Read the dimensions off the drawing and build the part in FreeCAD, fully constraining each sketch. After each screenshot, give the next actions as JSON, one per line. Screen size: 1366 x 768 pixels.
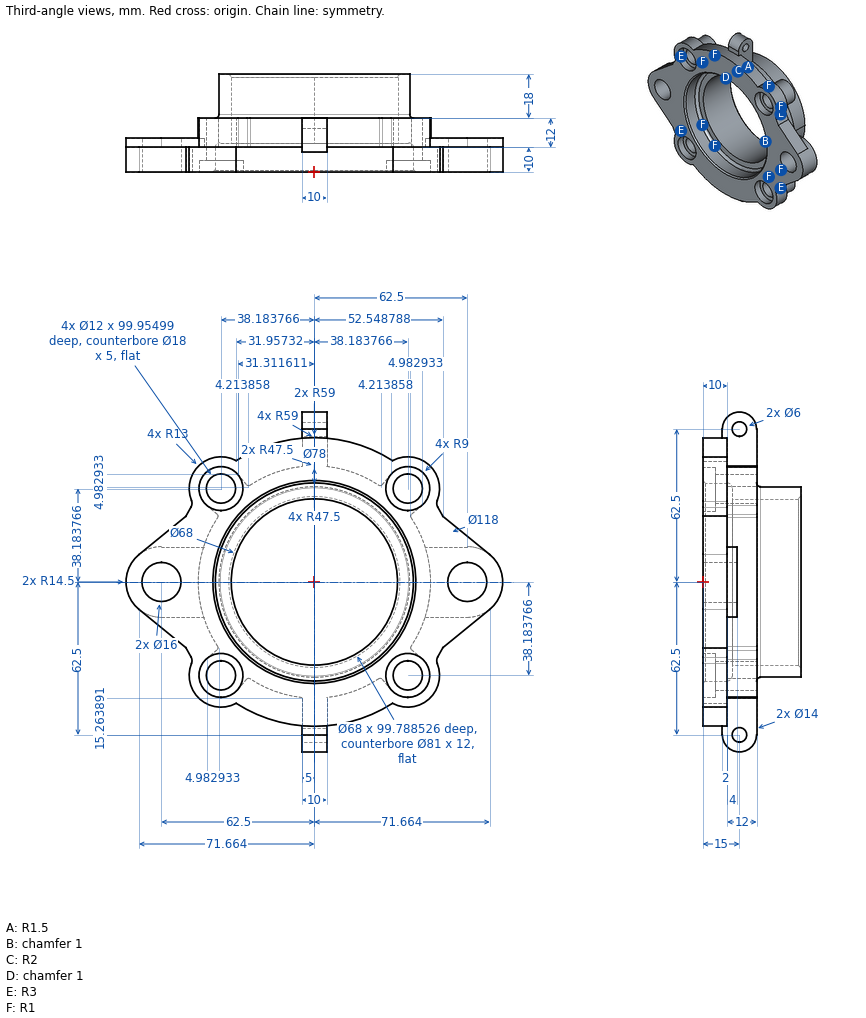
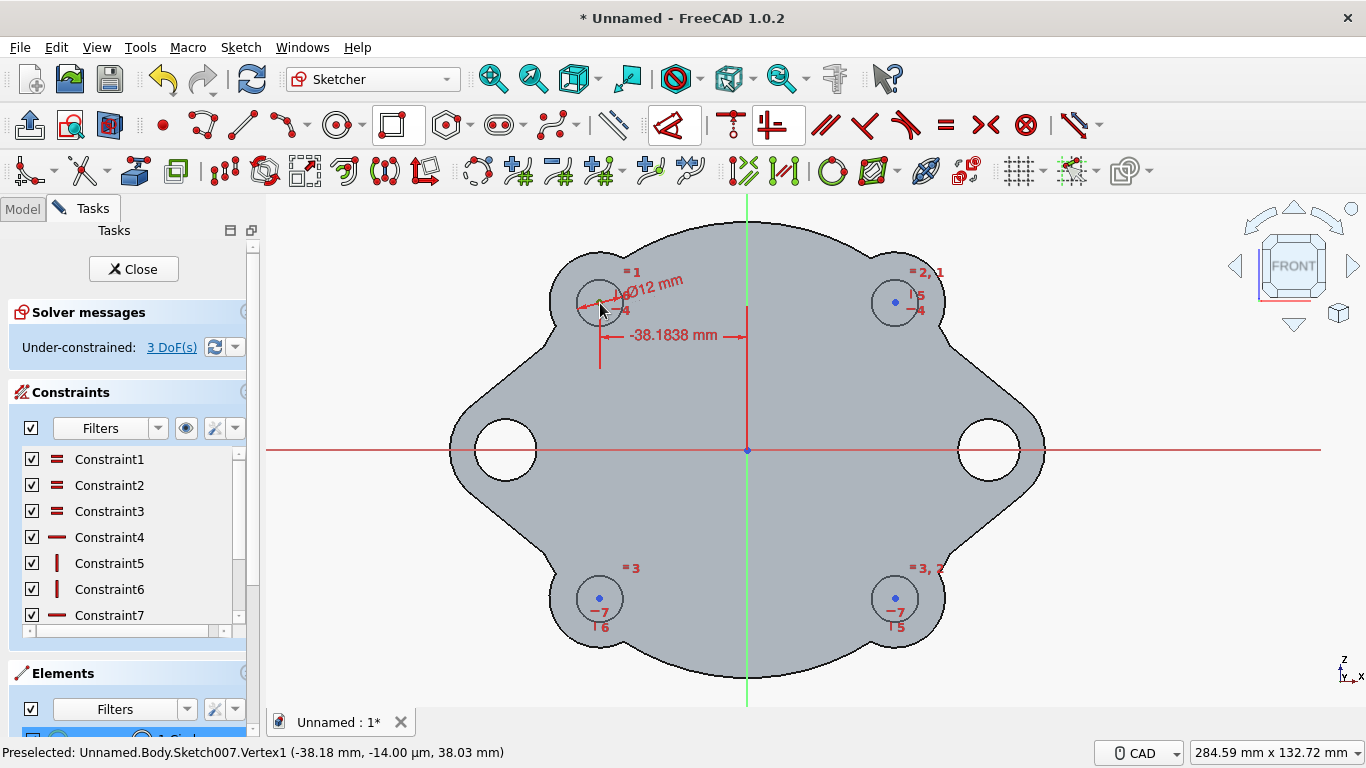
{"action": "left_click", "coordinate": [696, 126]}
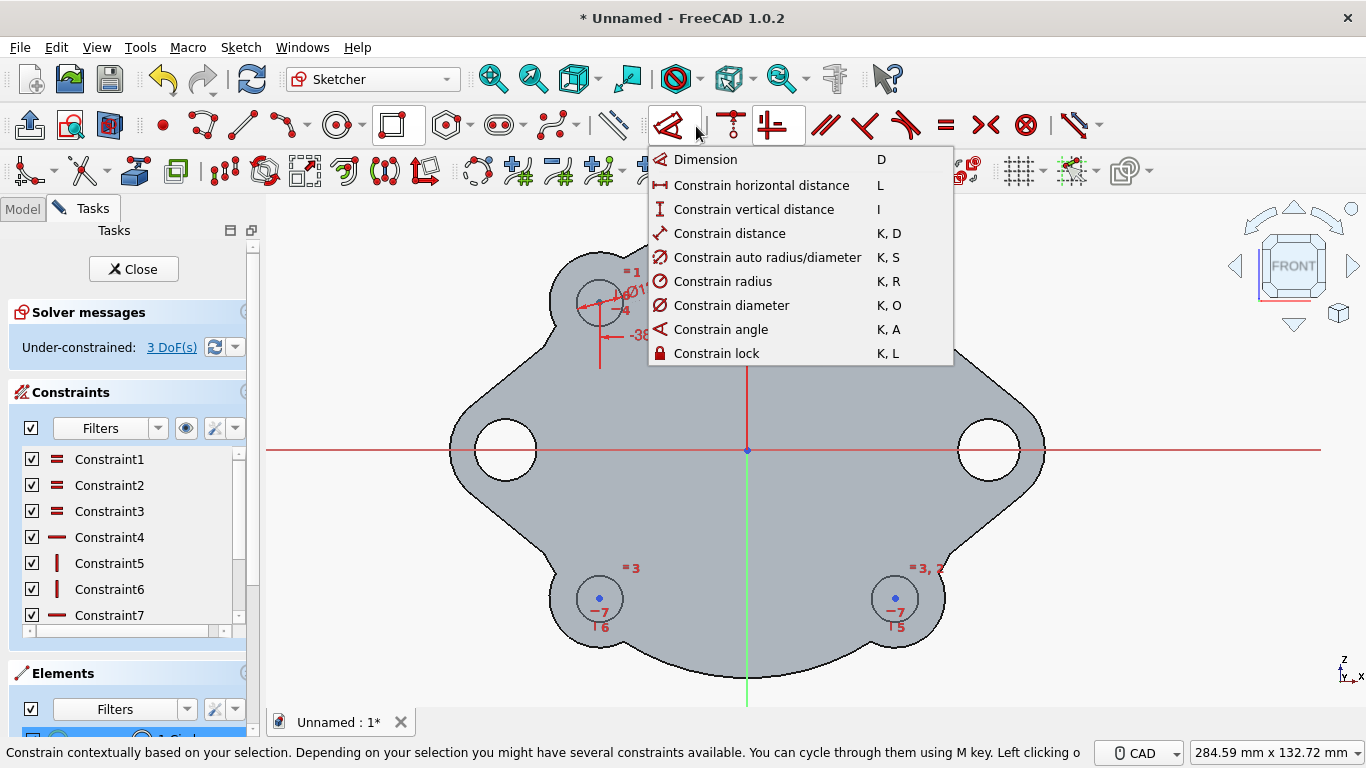
{"action": "left_click", "coordinate": [801, 209]}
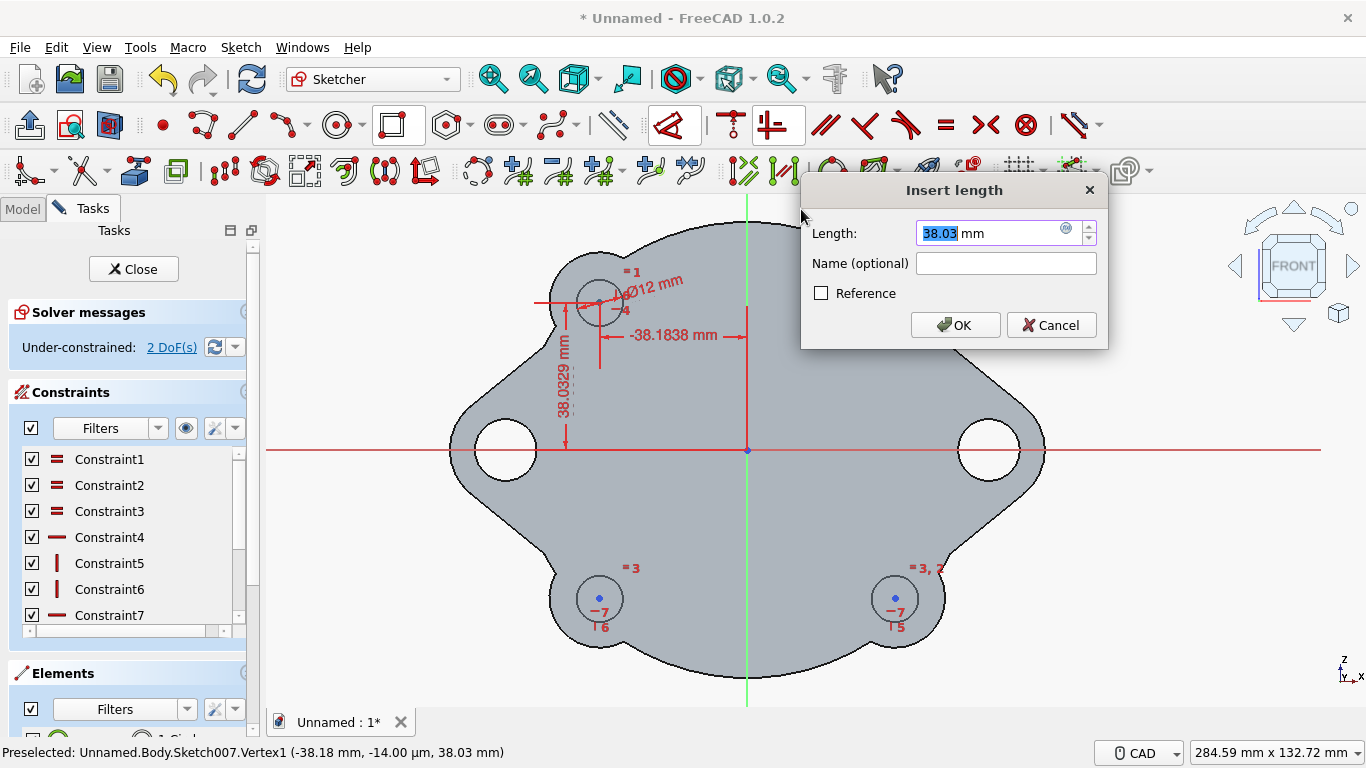
{"action": "type", "text": "38.183766"}
{"action": "key", "text": "Return"}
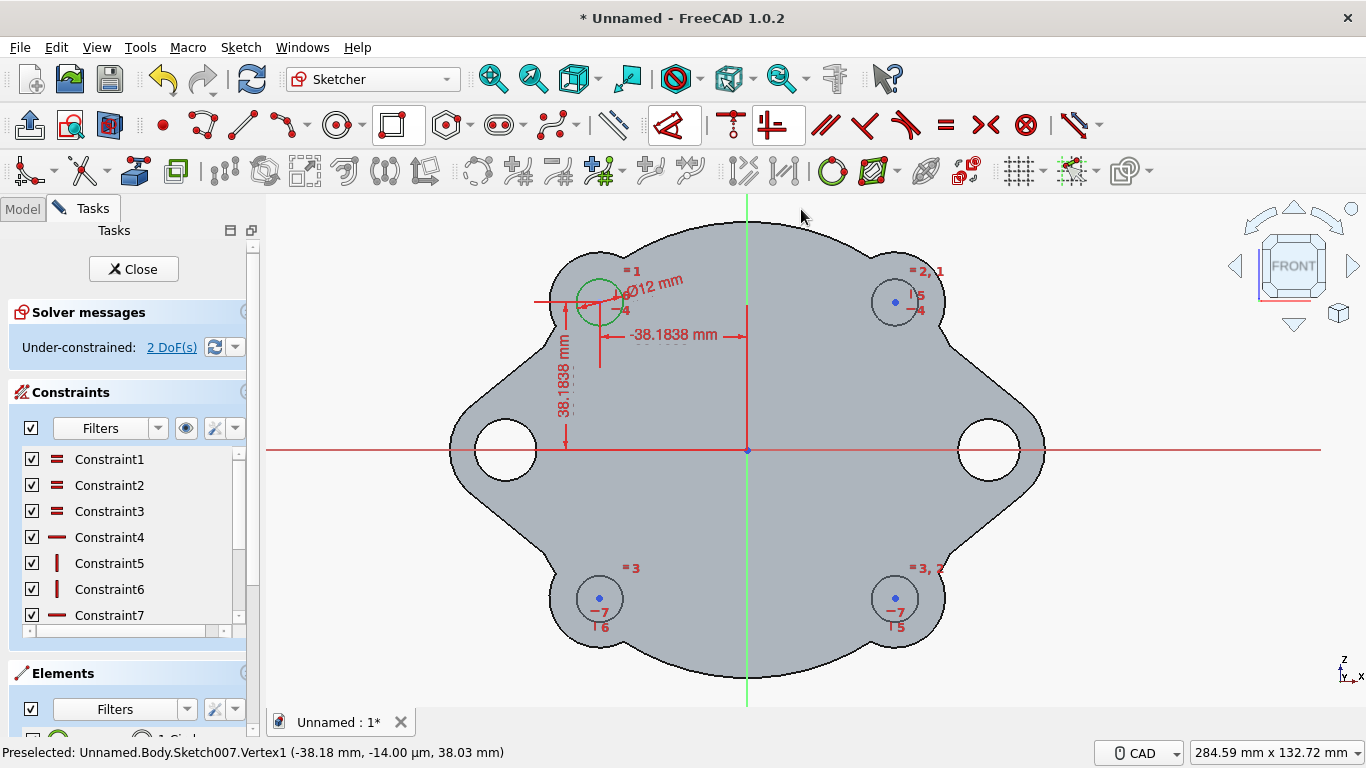
{"action": "left_click", "coordinate": [895, 302]}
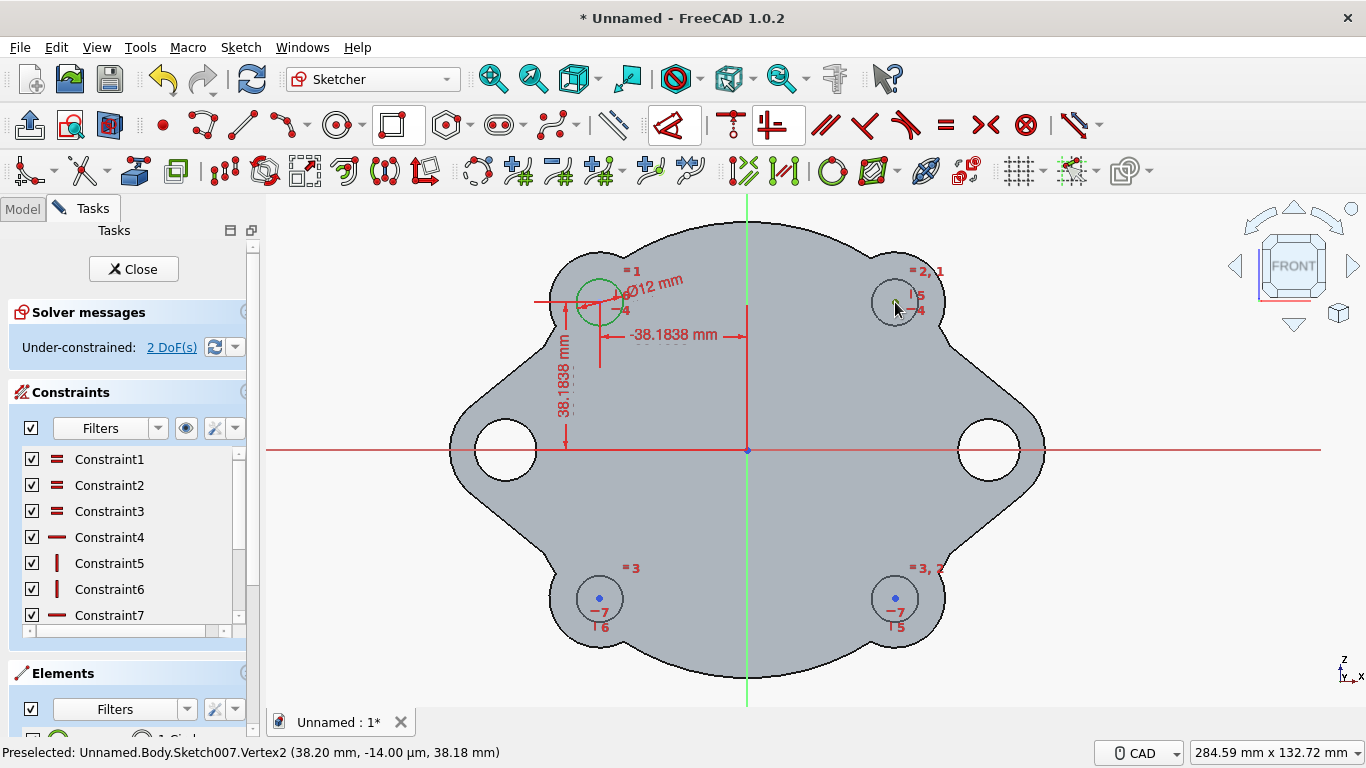
{"action": "left_click", "coordinate": [696, 126]}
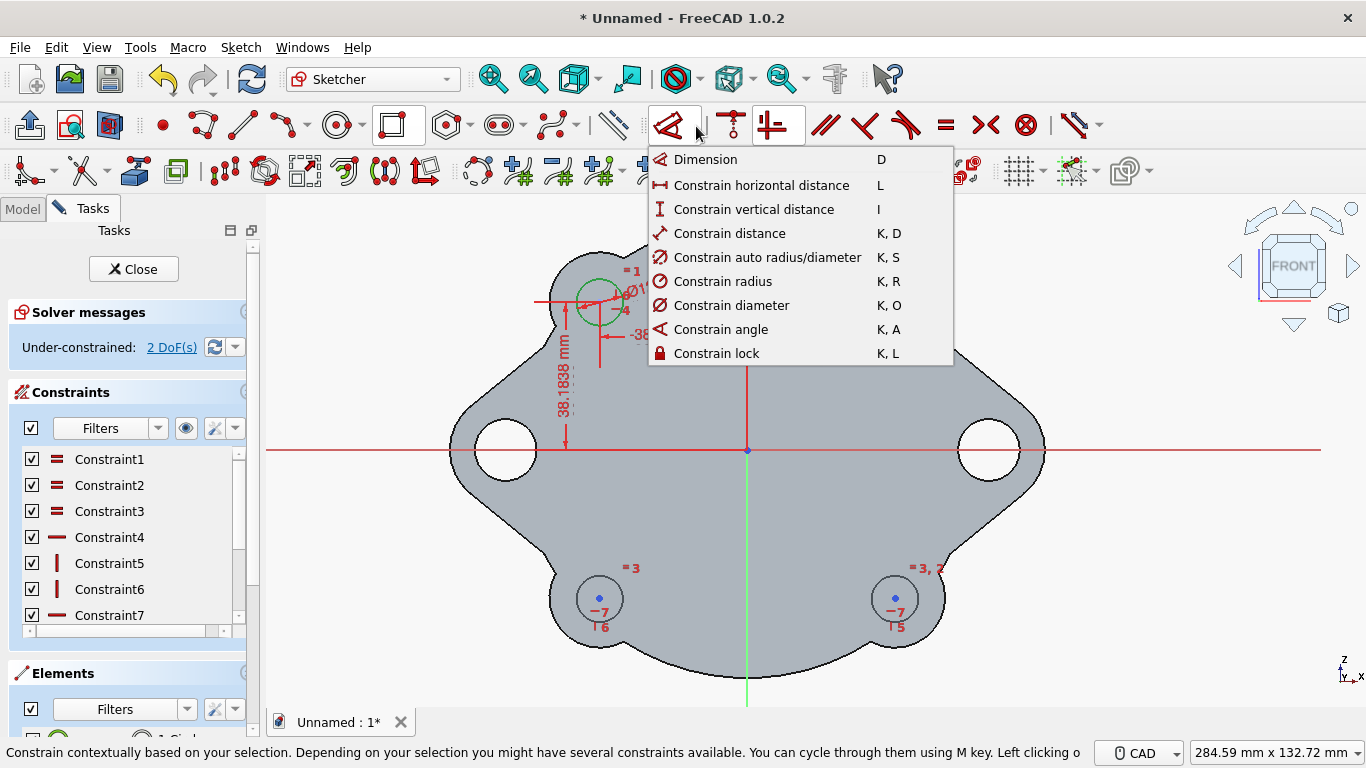
{"action": "left_click", "coordinate": [801, 185]}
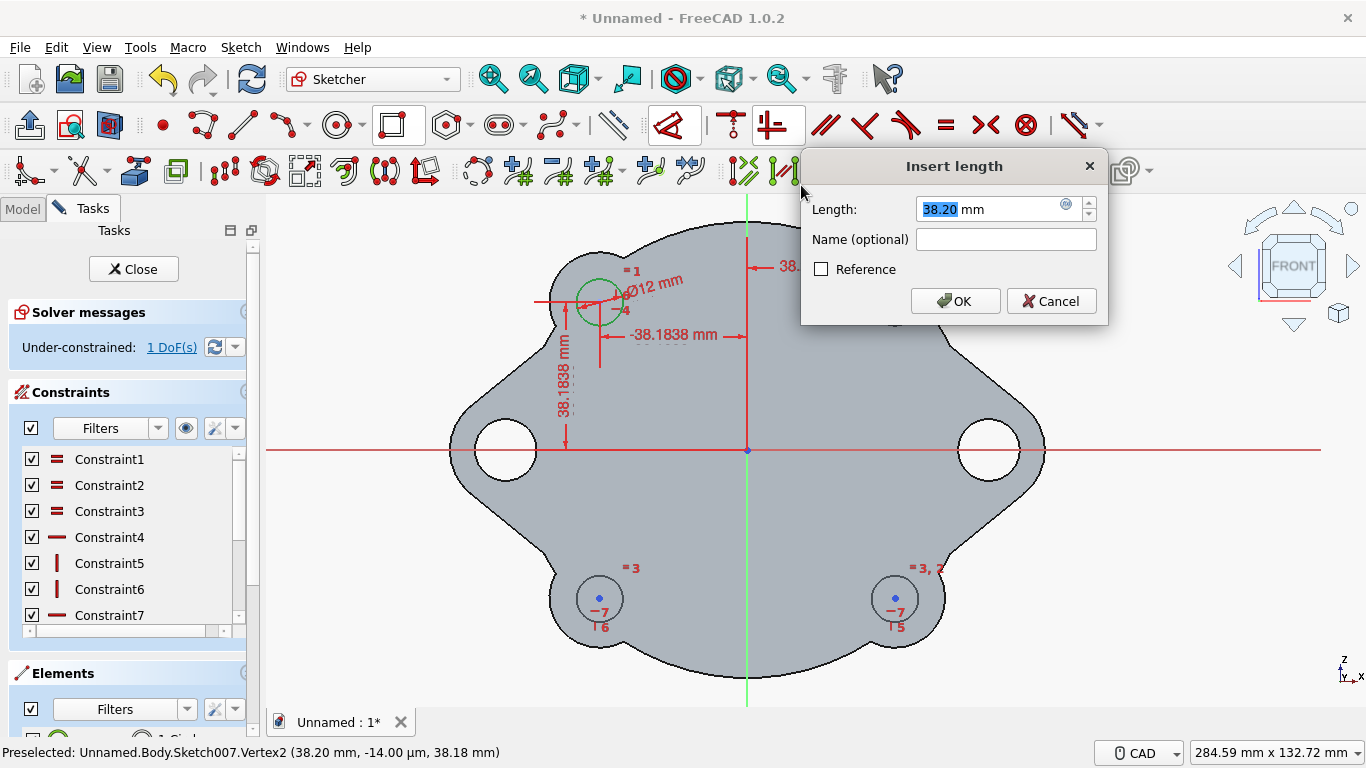
{"action": "type", "text": "38.183766"}
{"action": "key", "text": "Return"}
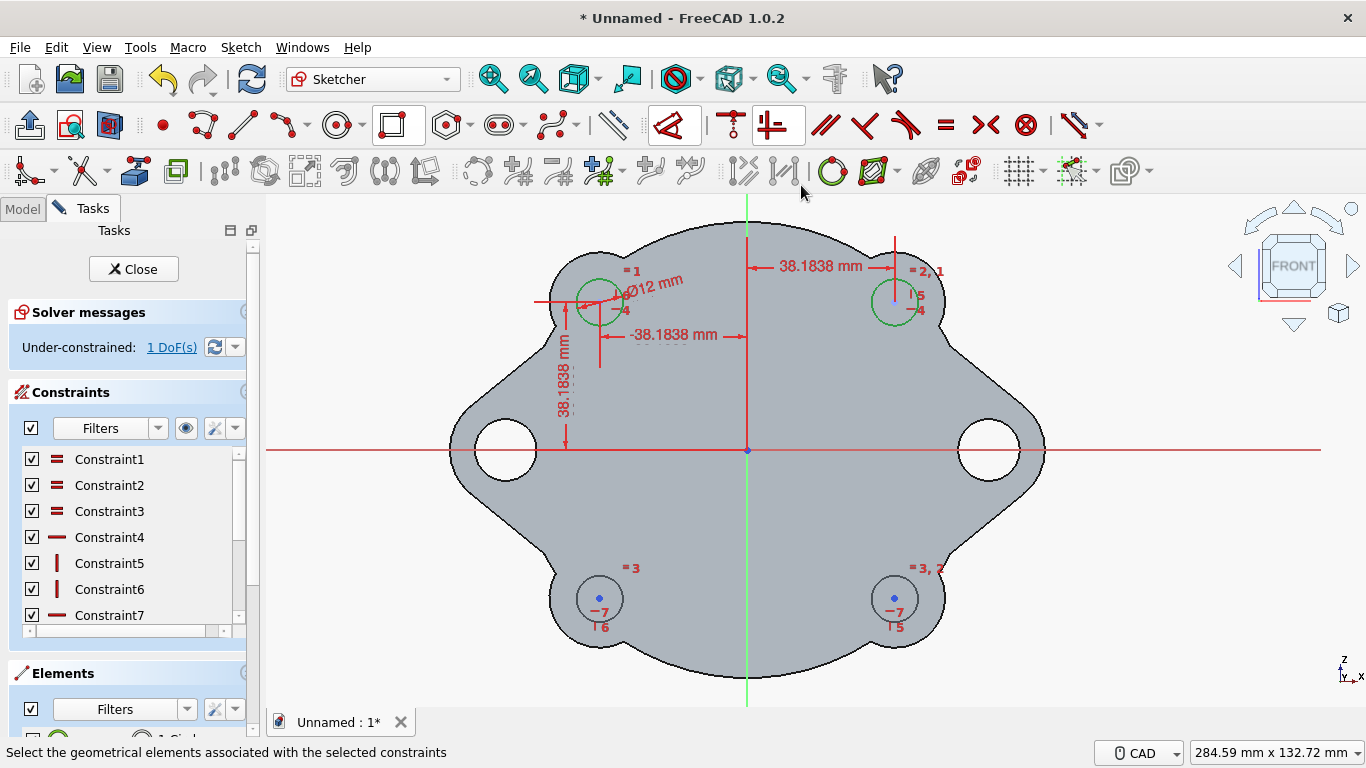
{"action": "left_click", "coordinate": [895, 599]}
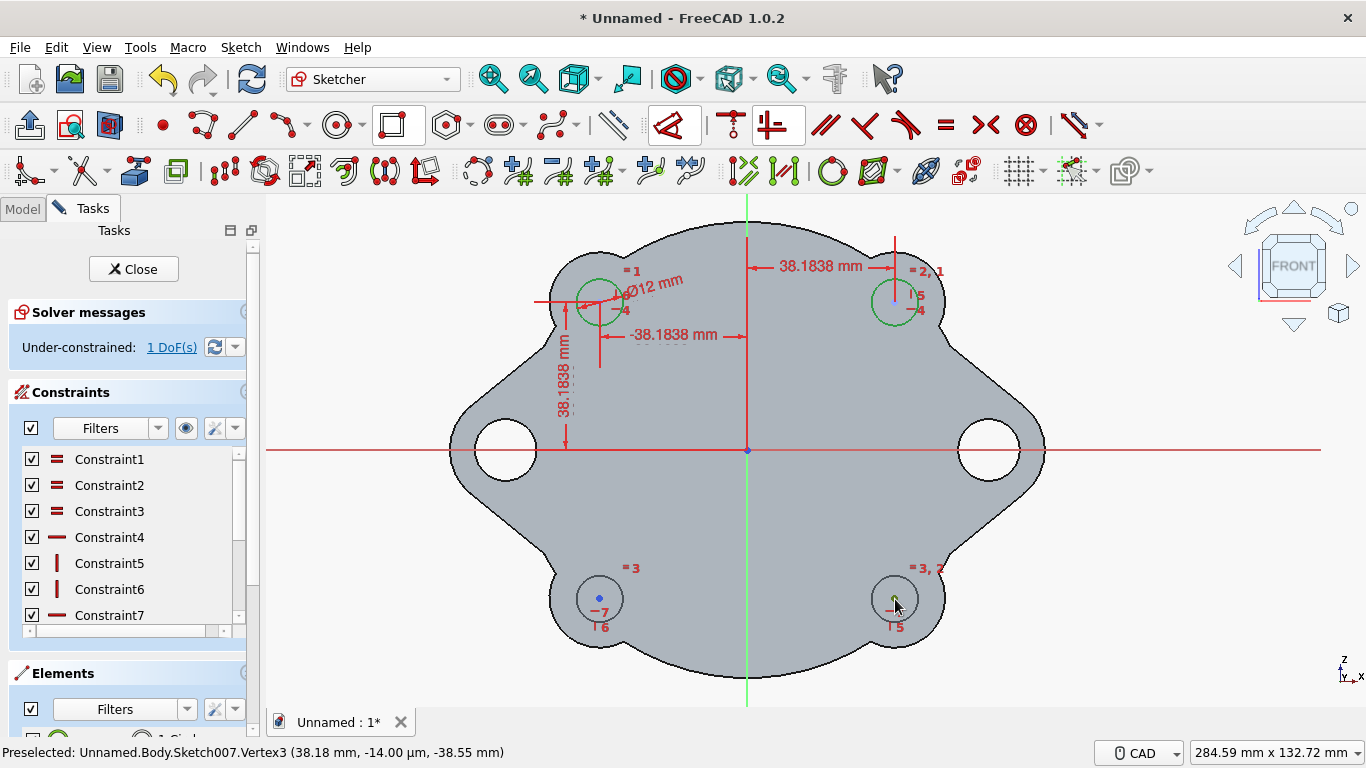
{"action": "left_click", "coordinate": [696, 126]}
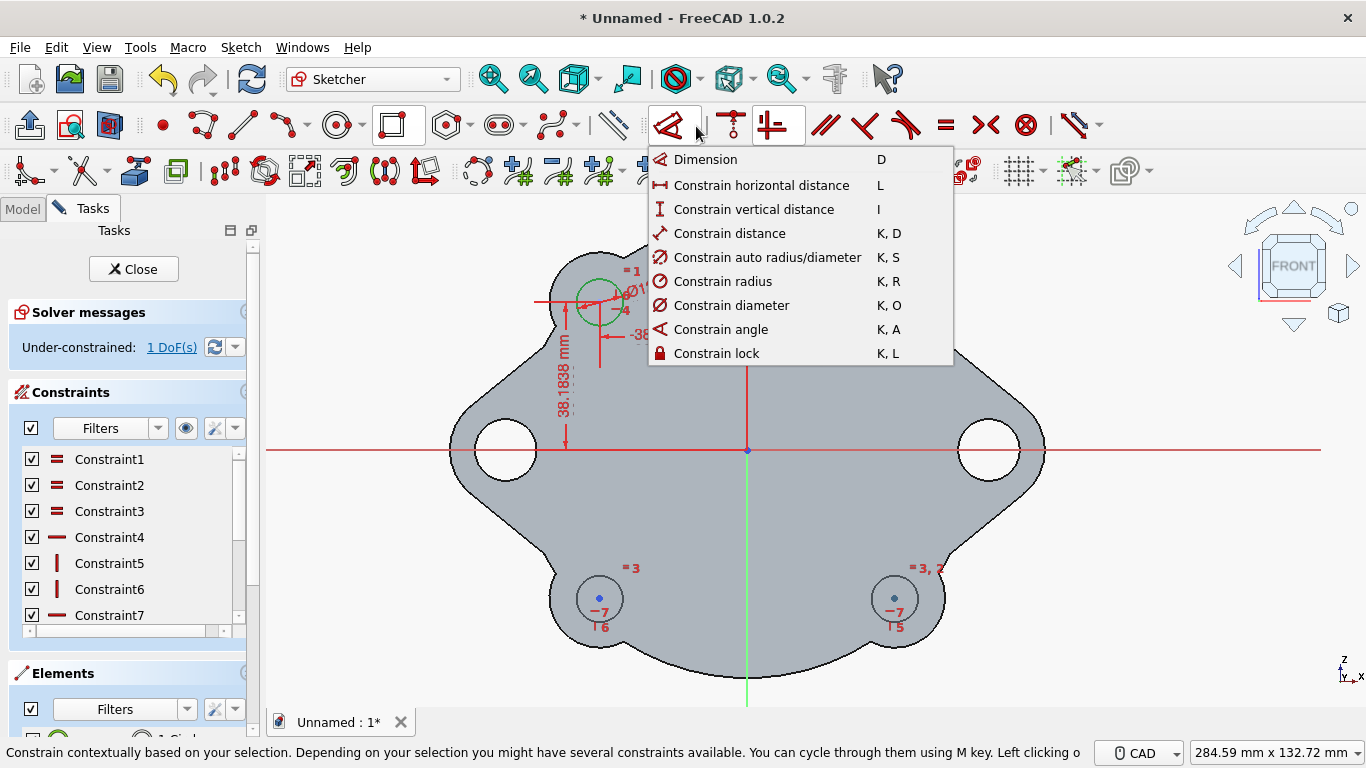
{"action": "left_click", "coordinate": [801, 209]}